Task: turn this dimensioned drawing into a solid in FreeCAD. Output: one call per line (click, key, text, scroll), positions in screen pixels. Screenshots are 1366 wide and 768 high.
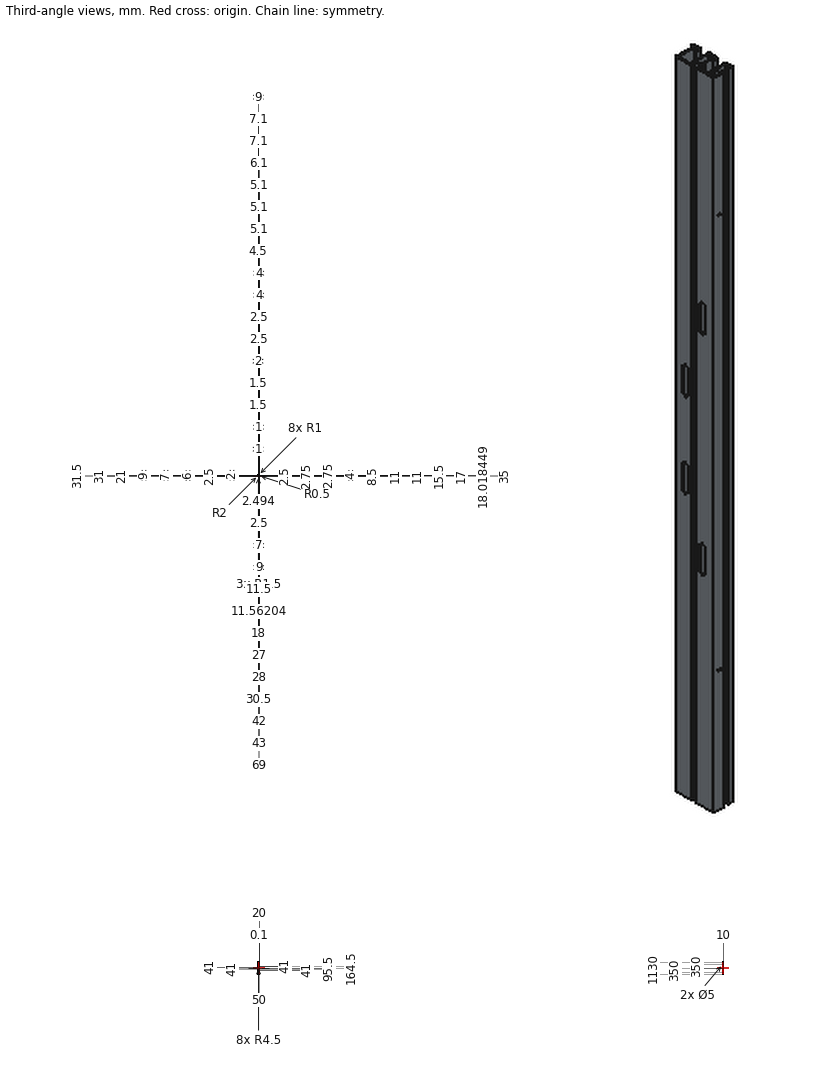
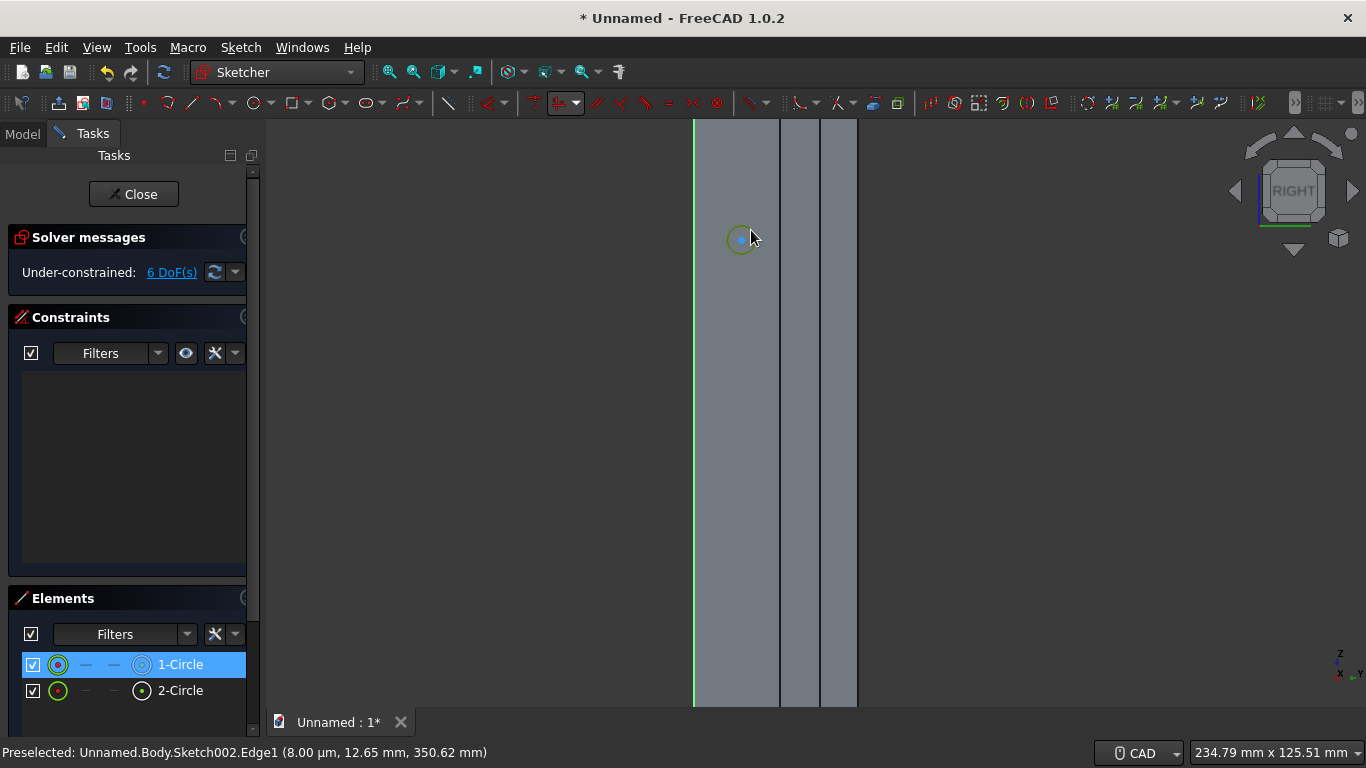
scroll(750, 231, down, 11)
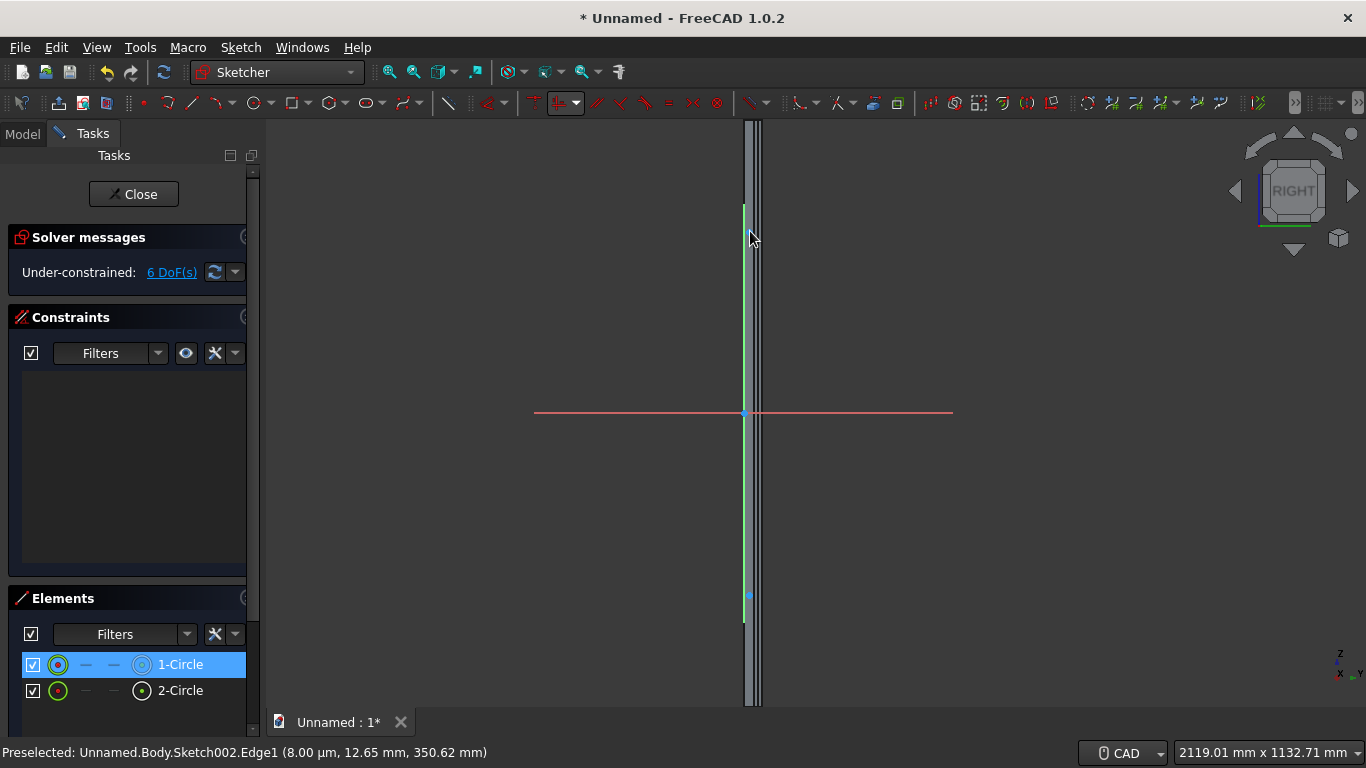
scroll(751, 595, up, 12)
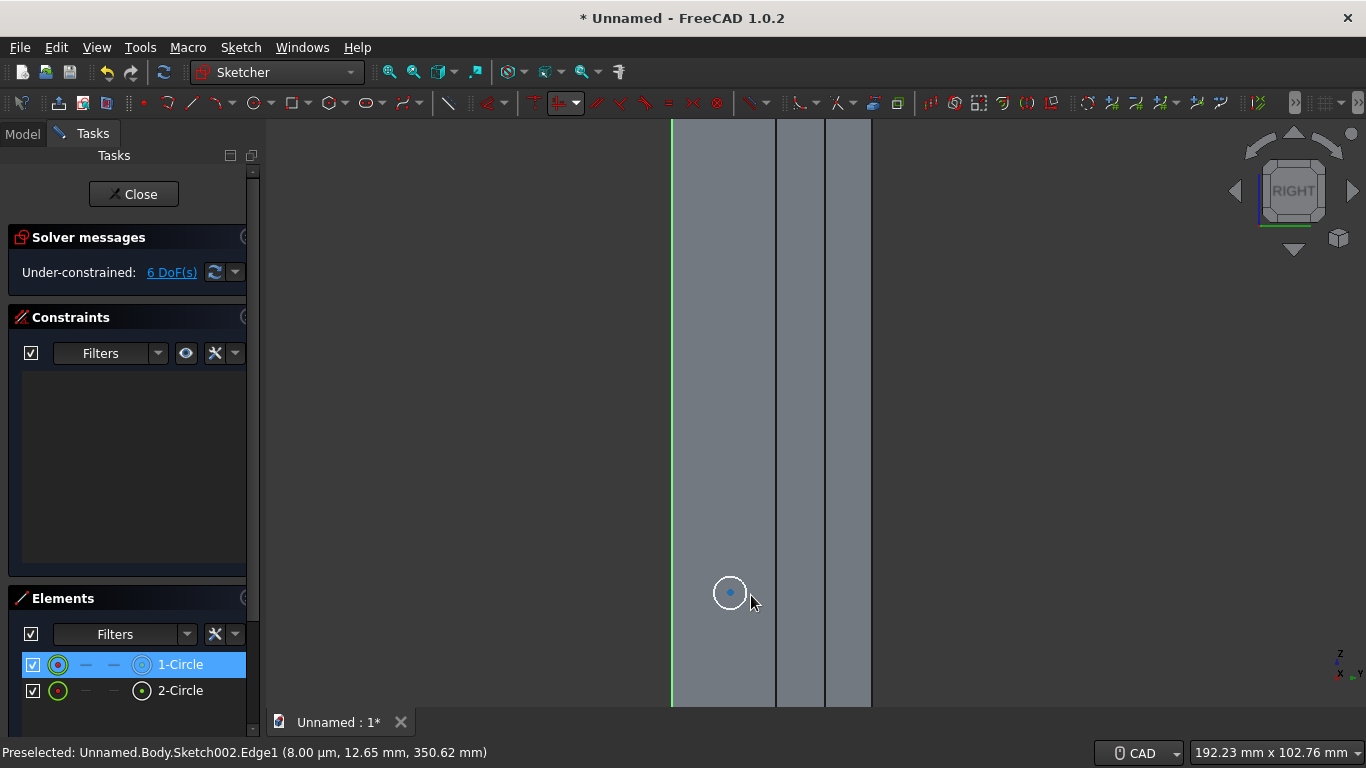
click(742, 581)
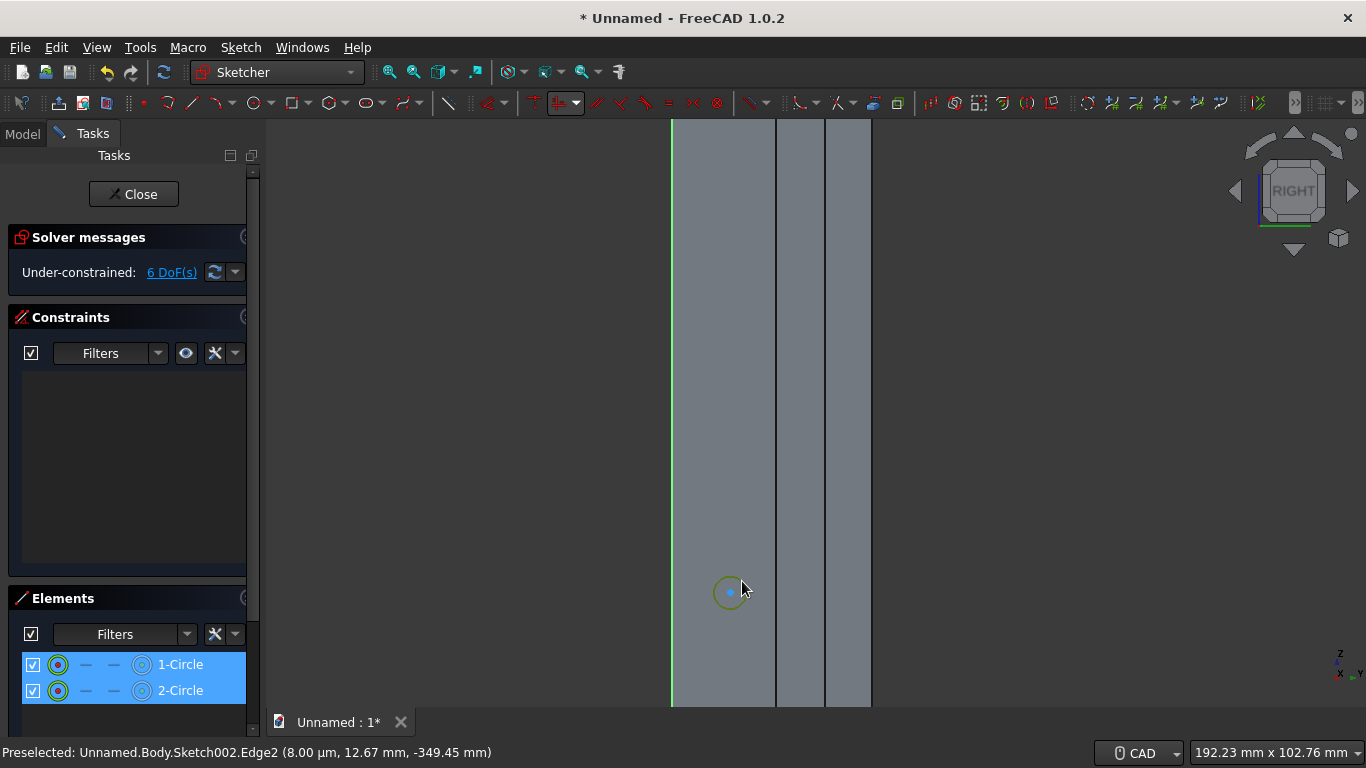
click(670, 104)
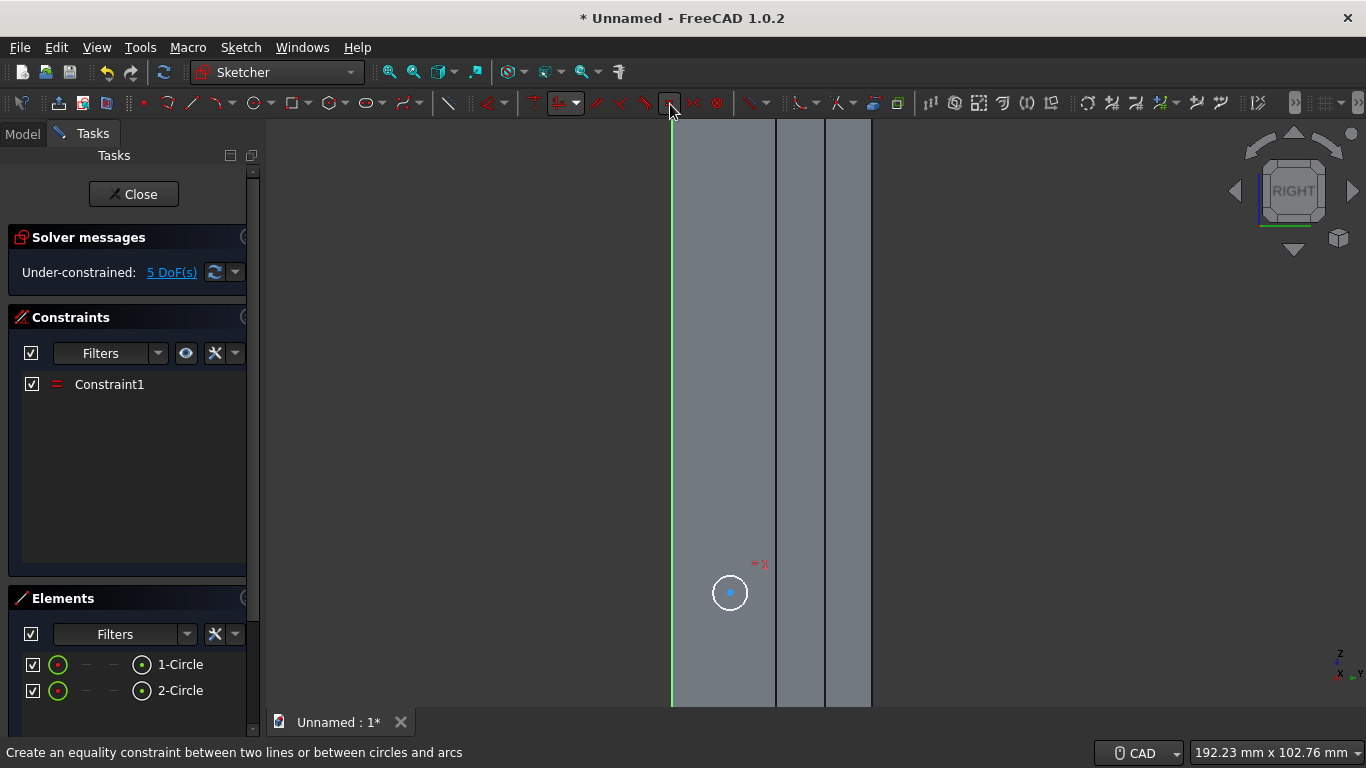
scroll(751, 595, down, 12)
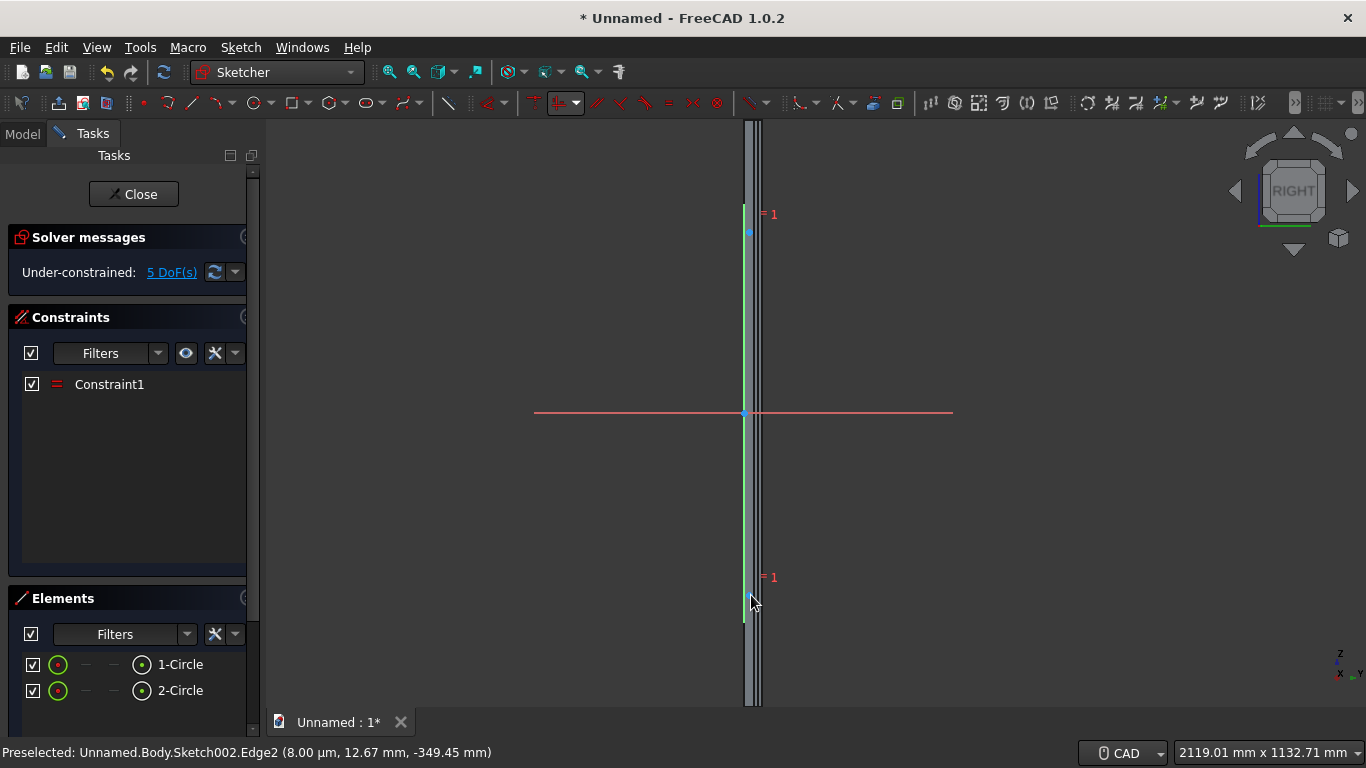
click(749, 232)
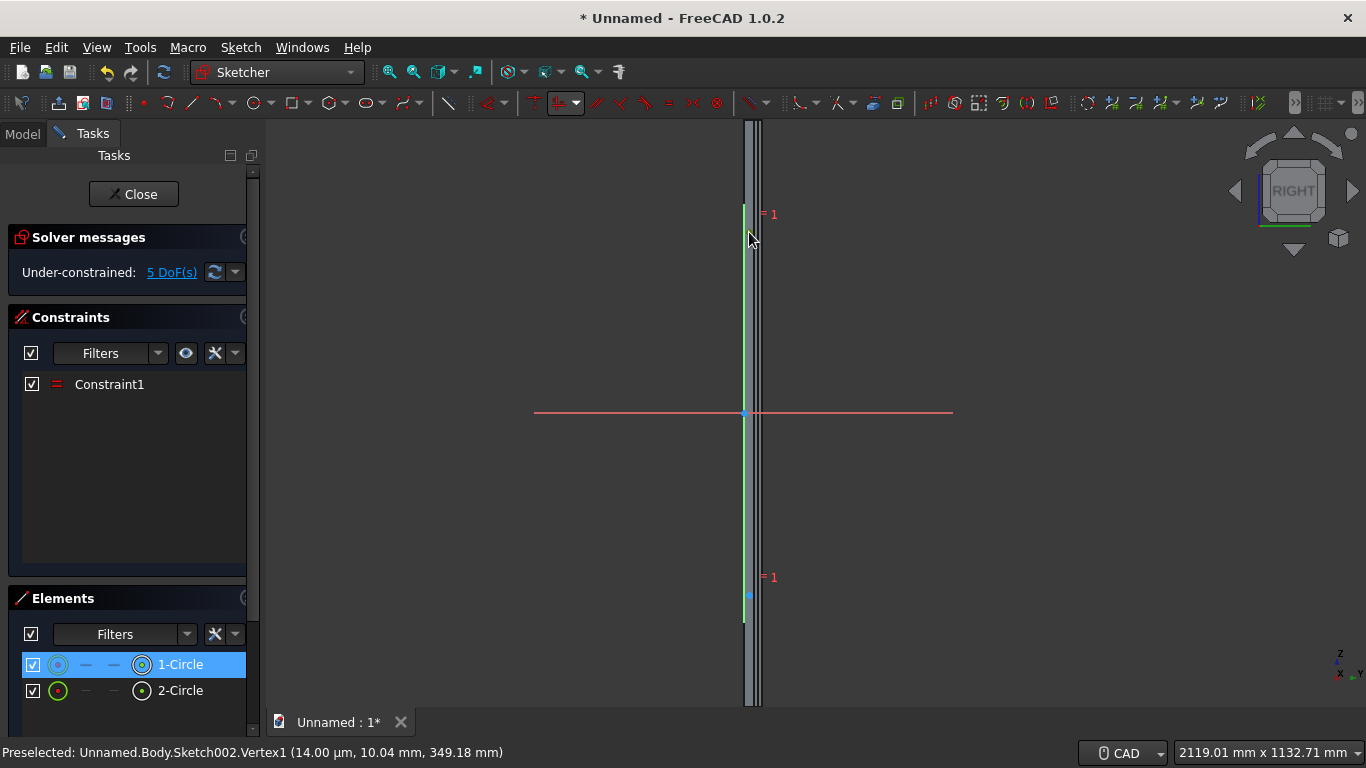
click(750, 596)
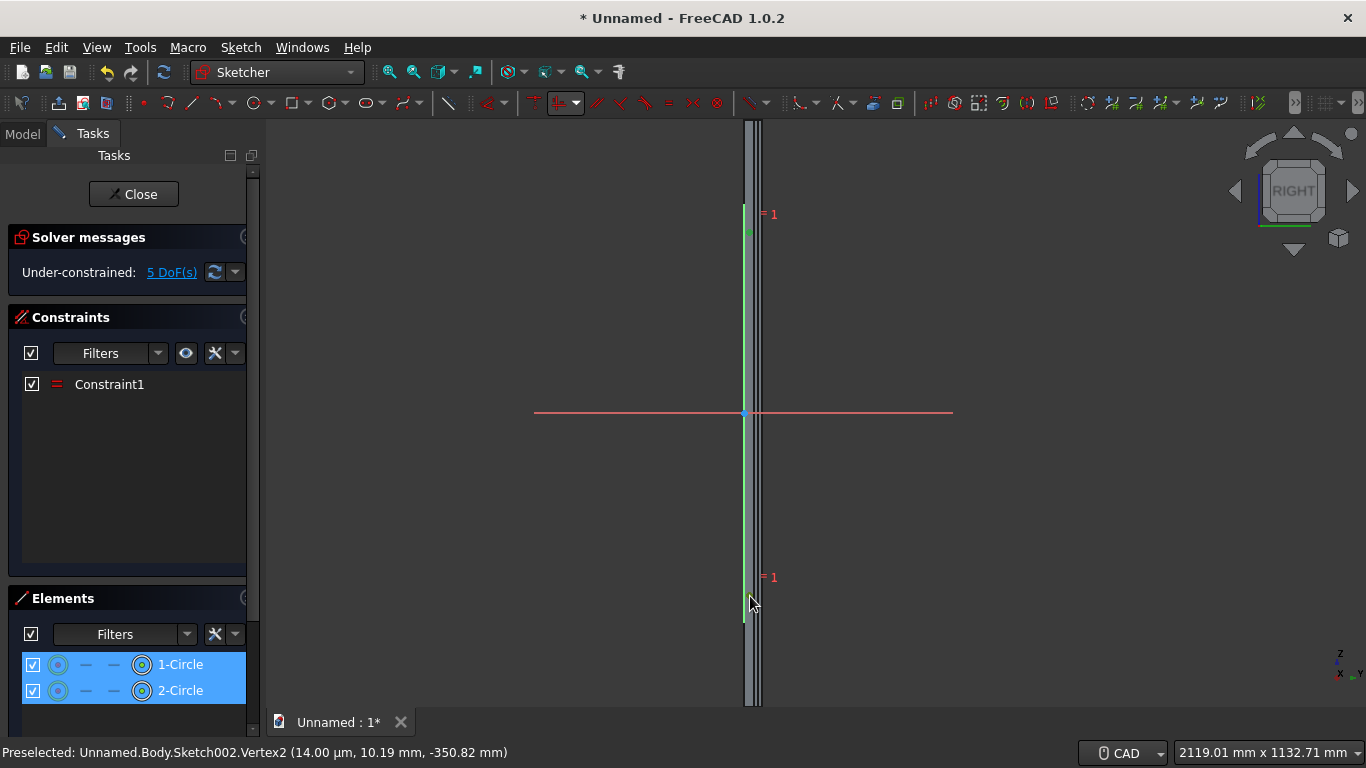
key(v)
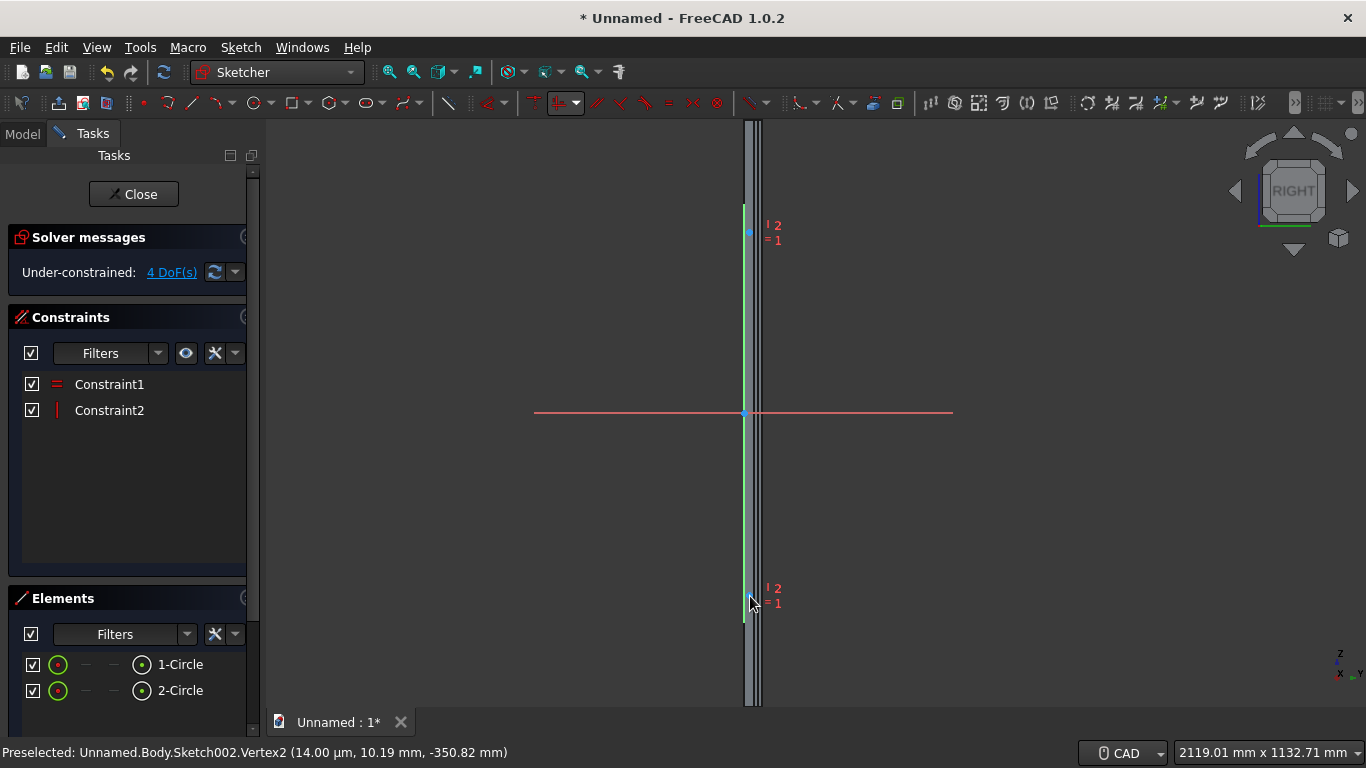
click(488, 104)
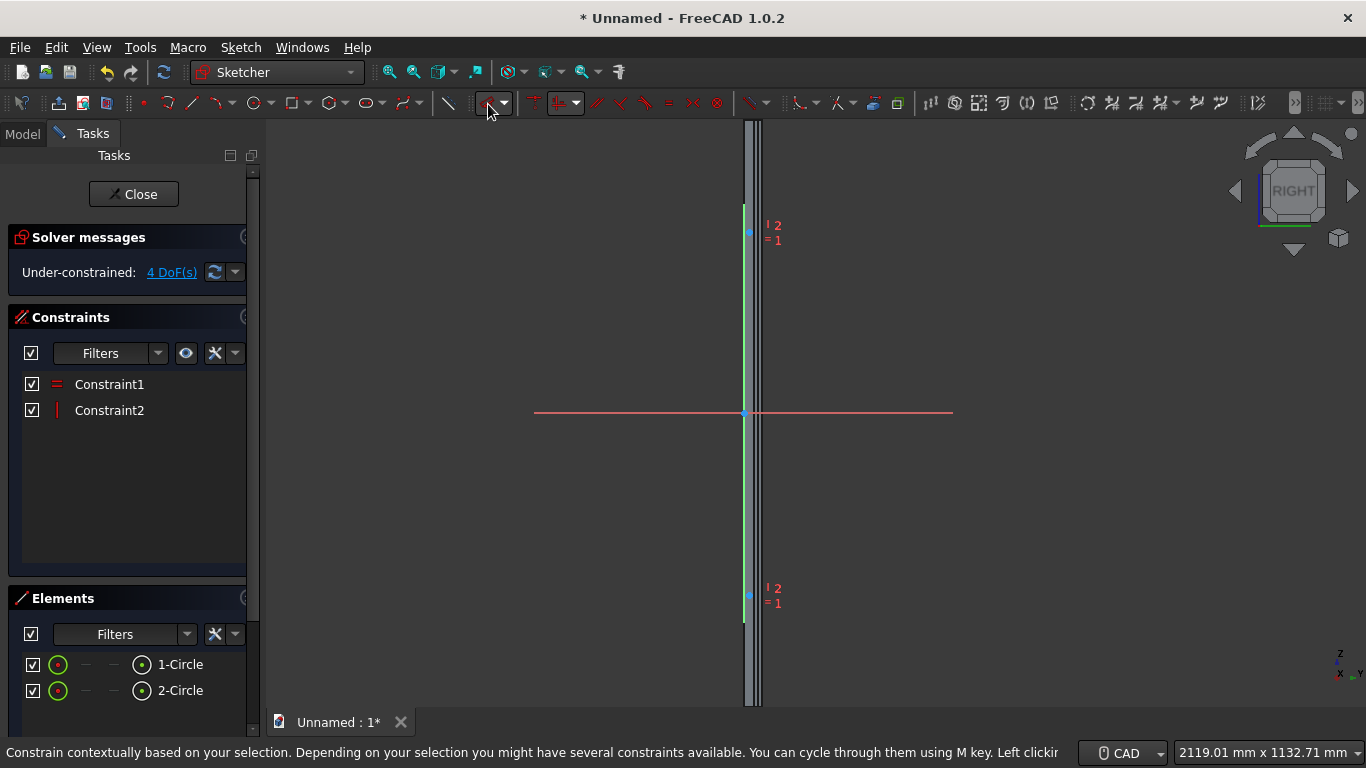
scroll(749, 234, up, 14)